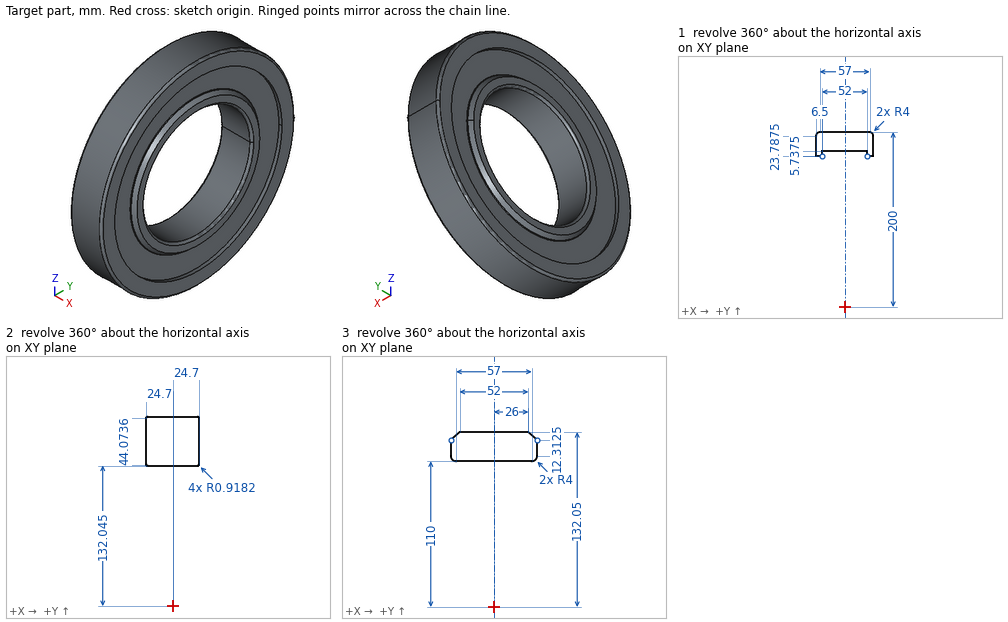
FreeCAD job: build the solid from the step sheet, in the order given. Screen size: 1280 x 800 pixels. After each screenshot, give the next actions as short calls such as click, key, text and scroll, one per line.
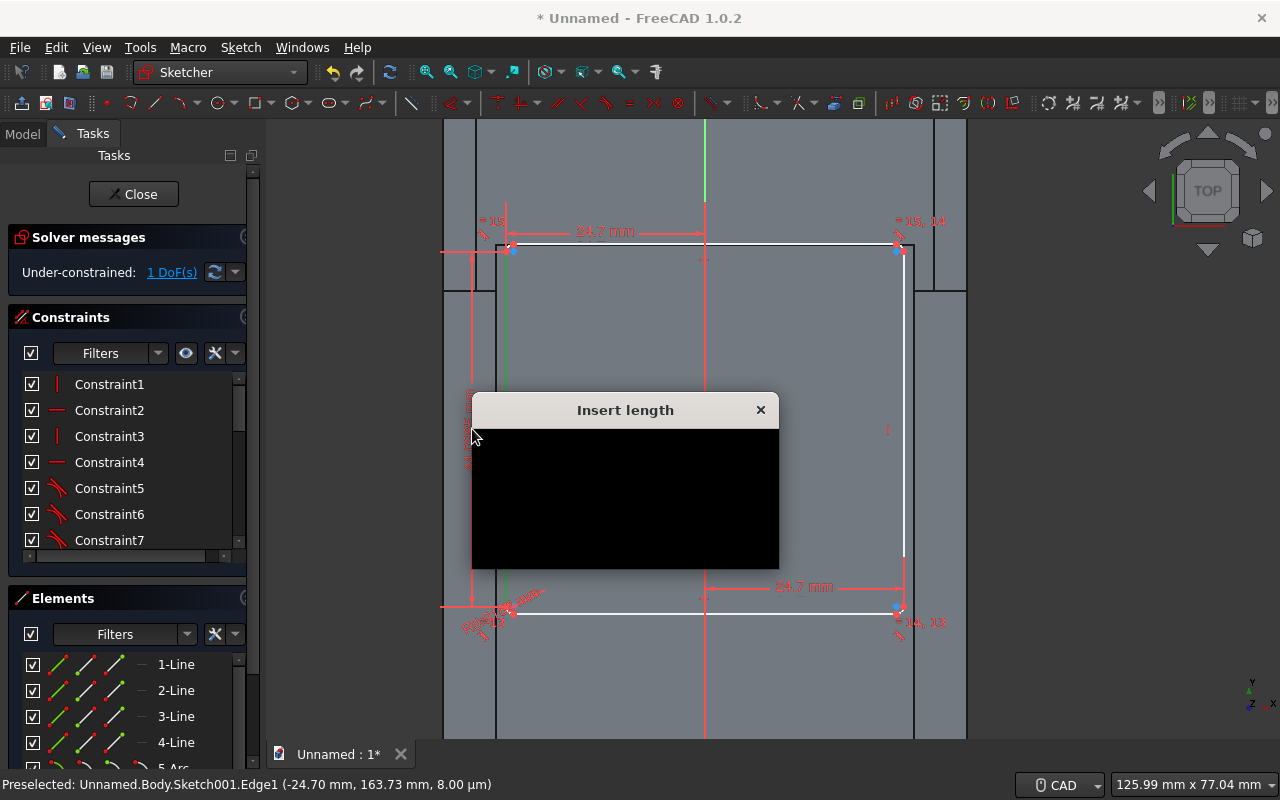
text(44.0736)
key(Return)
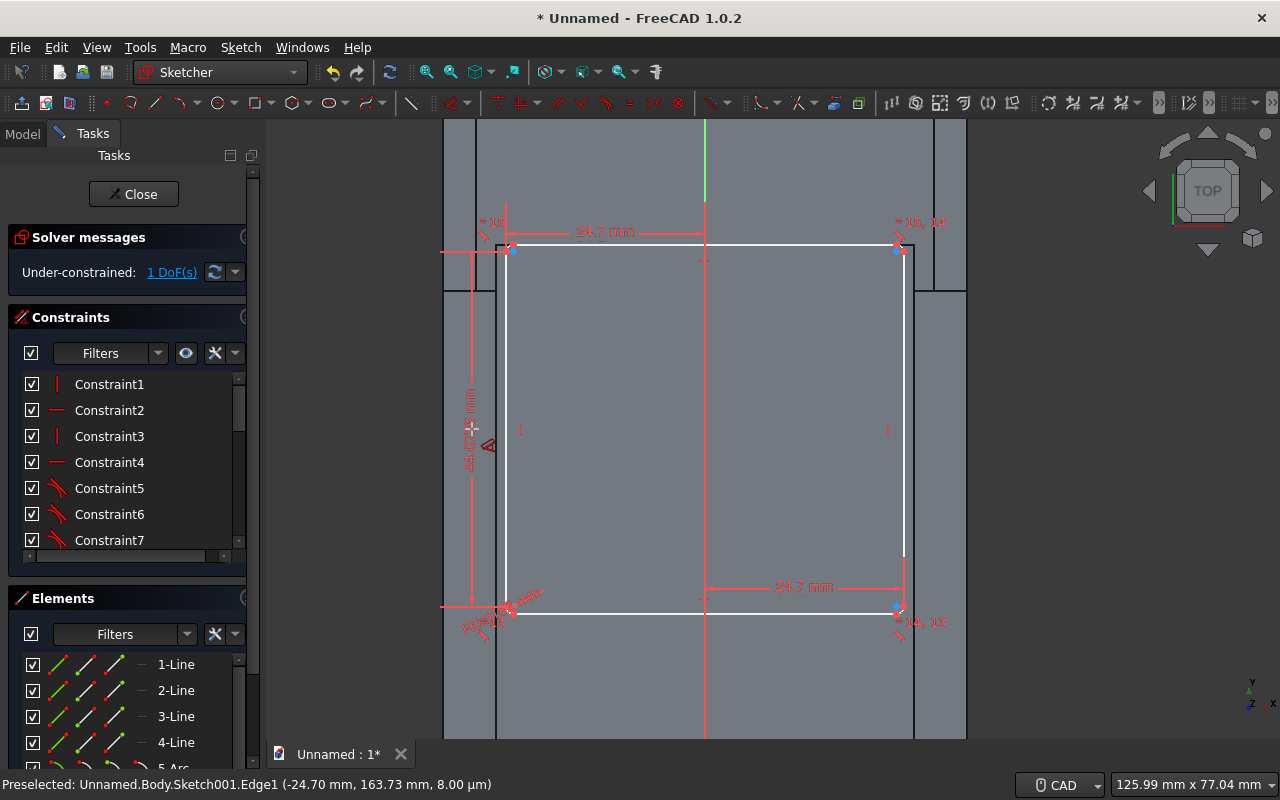
scroll(514, 614, up, 3)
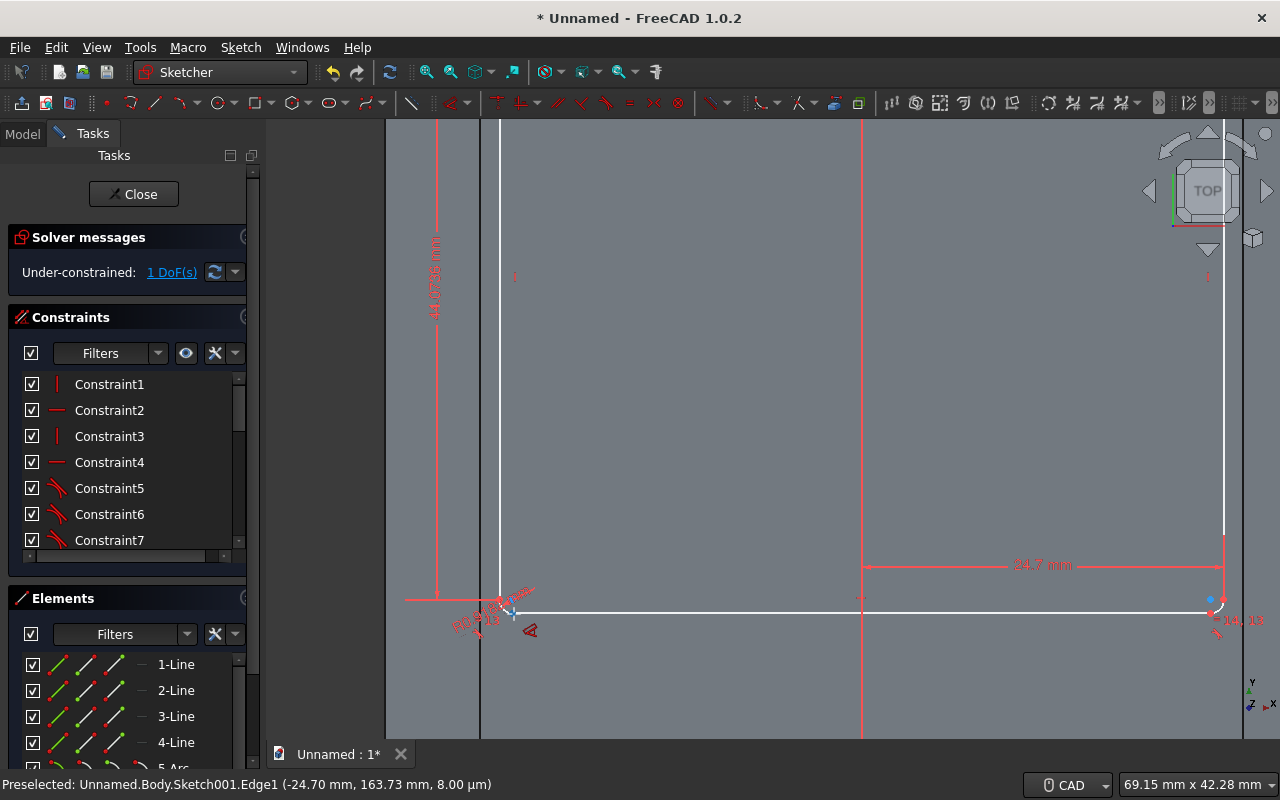
click(513, 613)
click(479, 662)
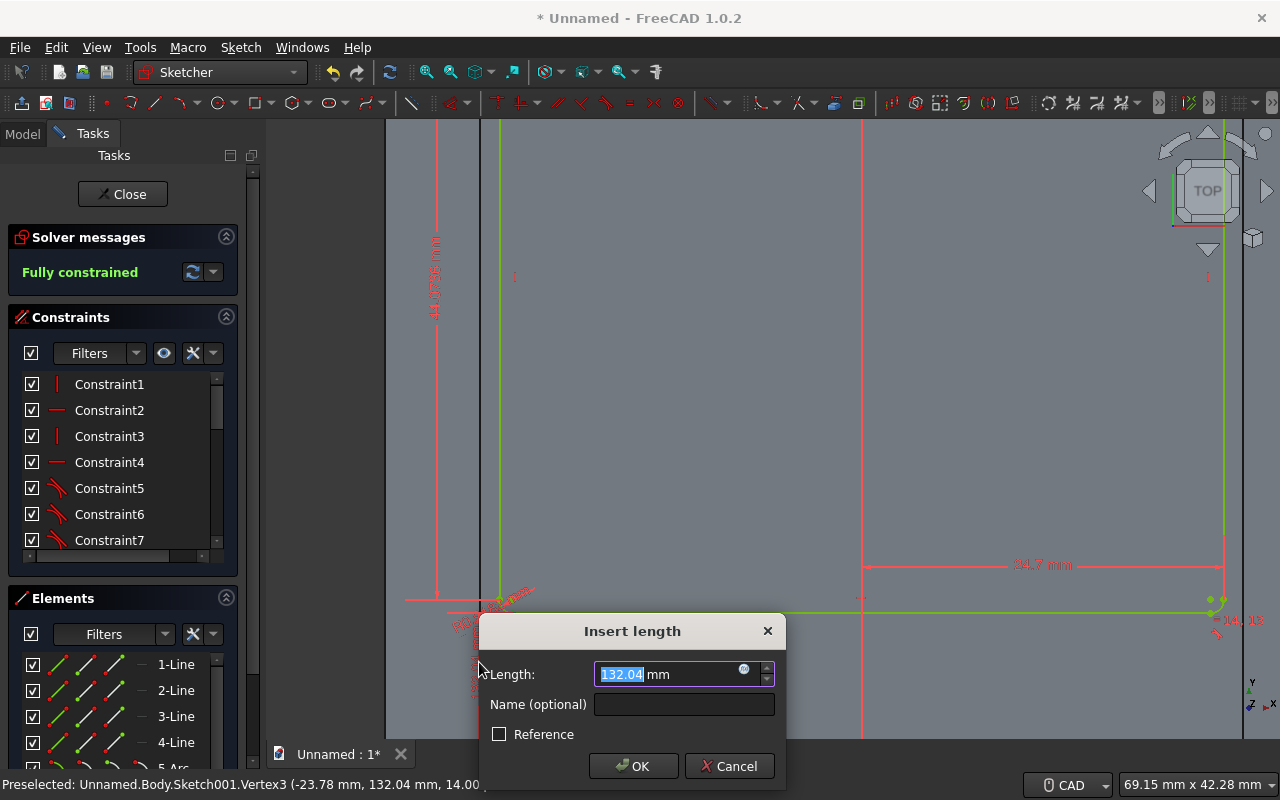
text(132.045)
key(Return)
key(Escape)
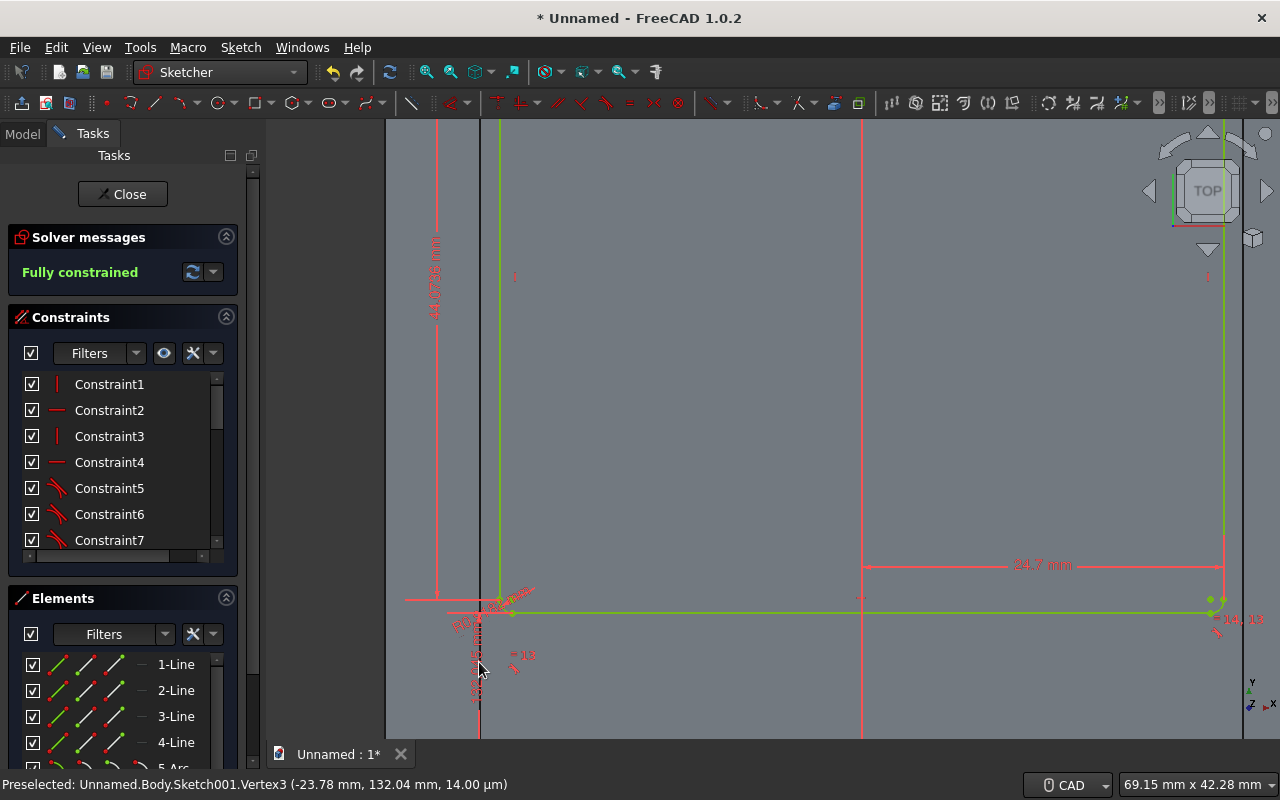
click(123, 194)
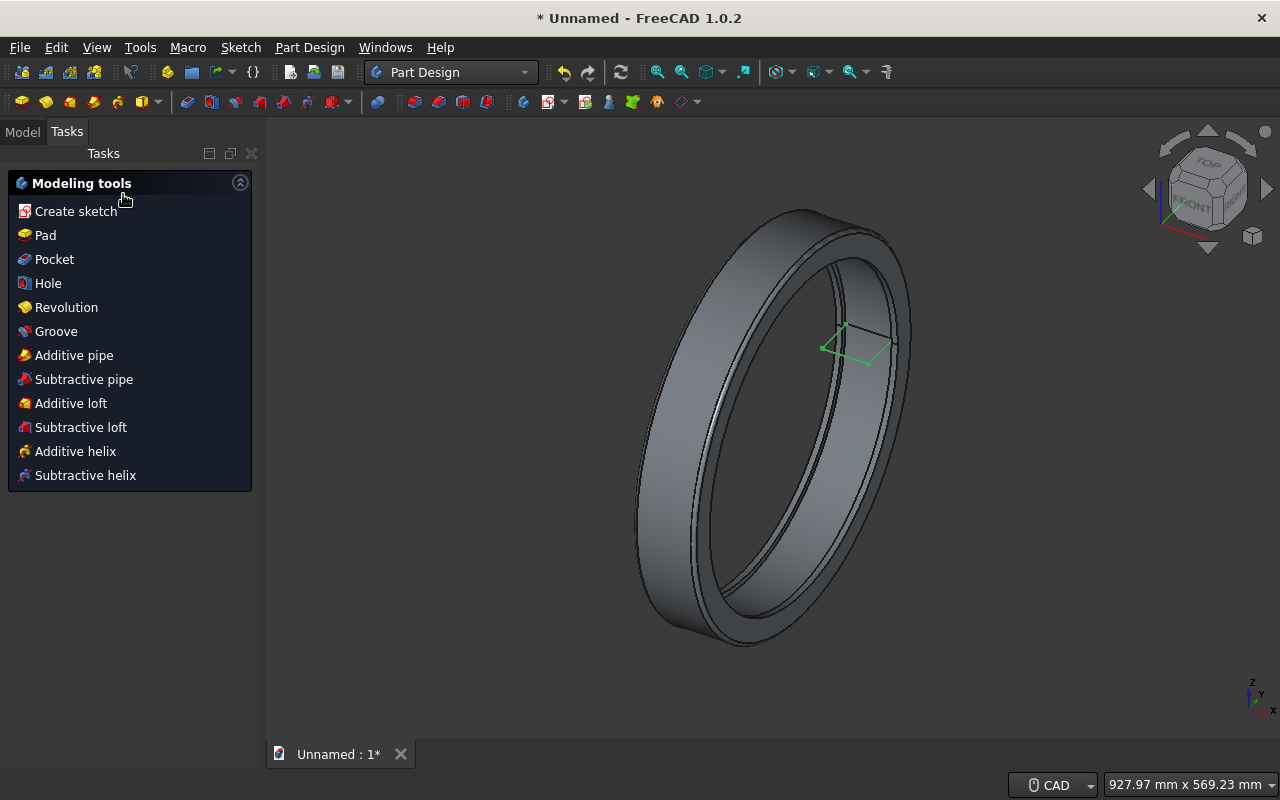
click(46, 102)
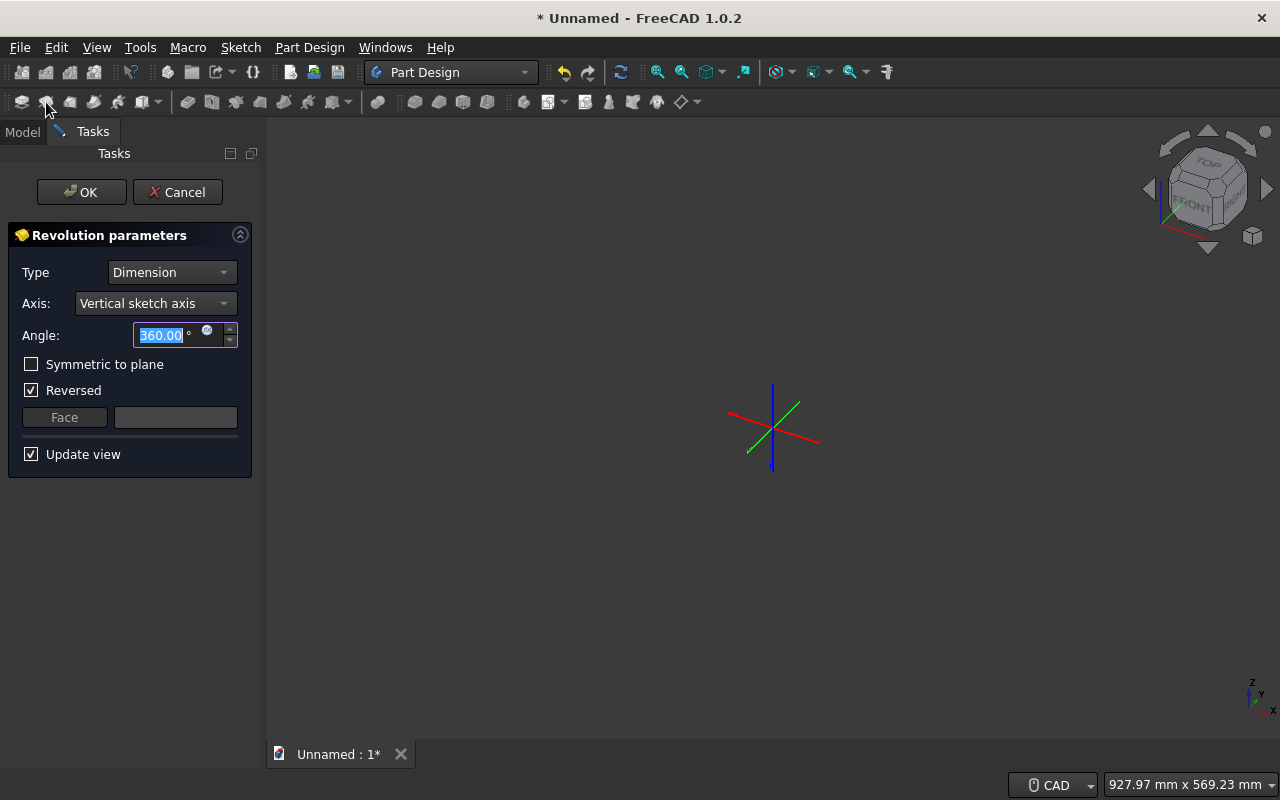
click(156, 304)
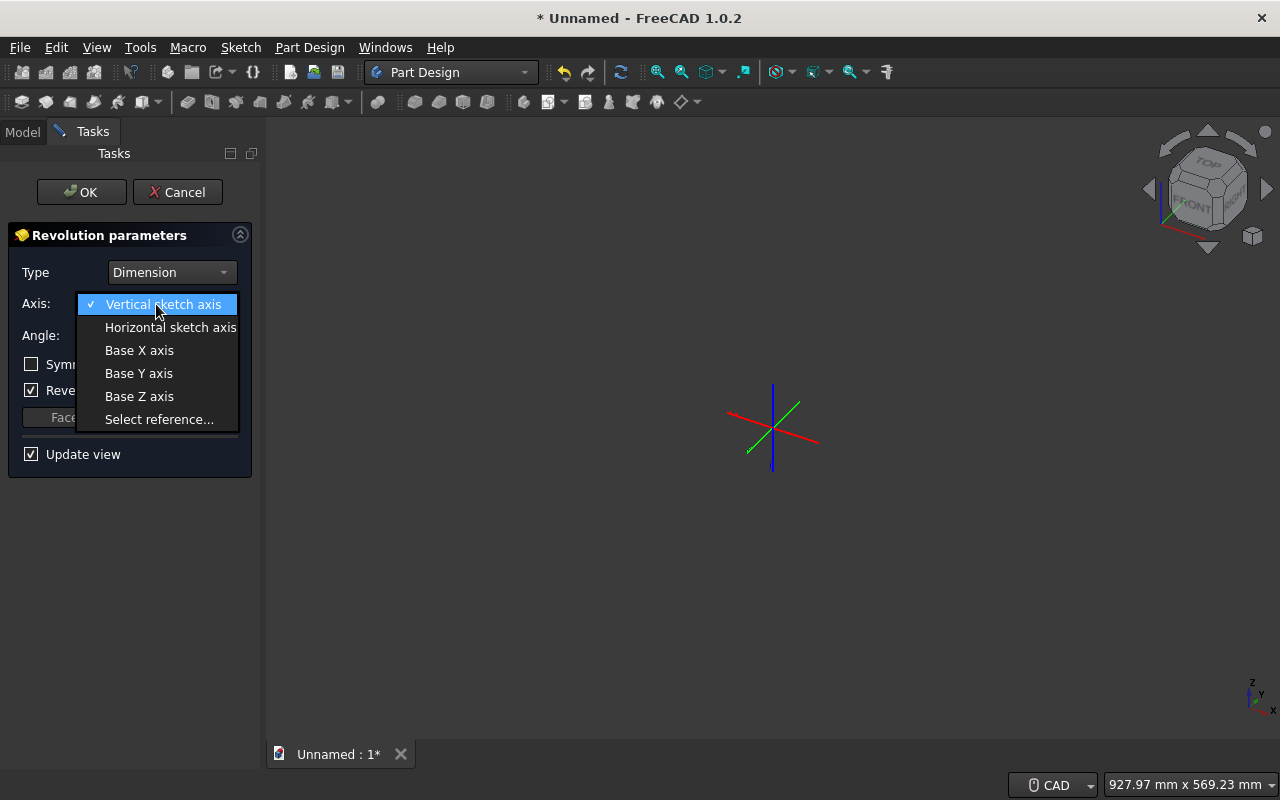
click(156, 328)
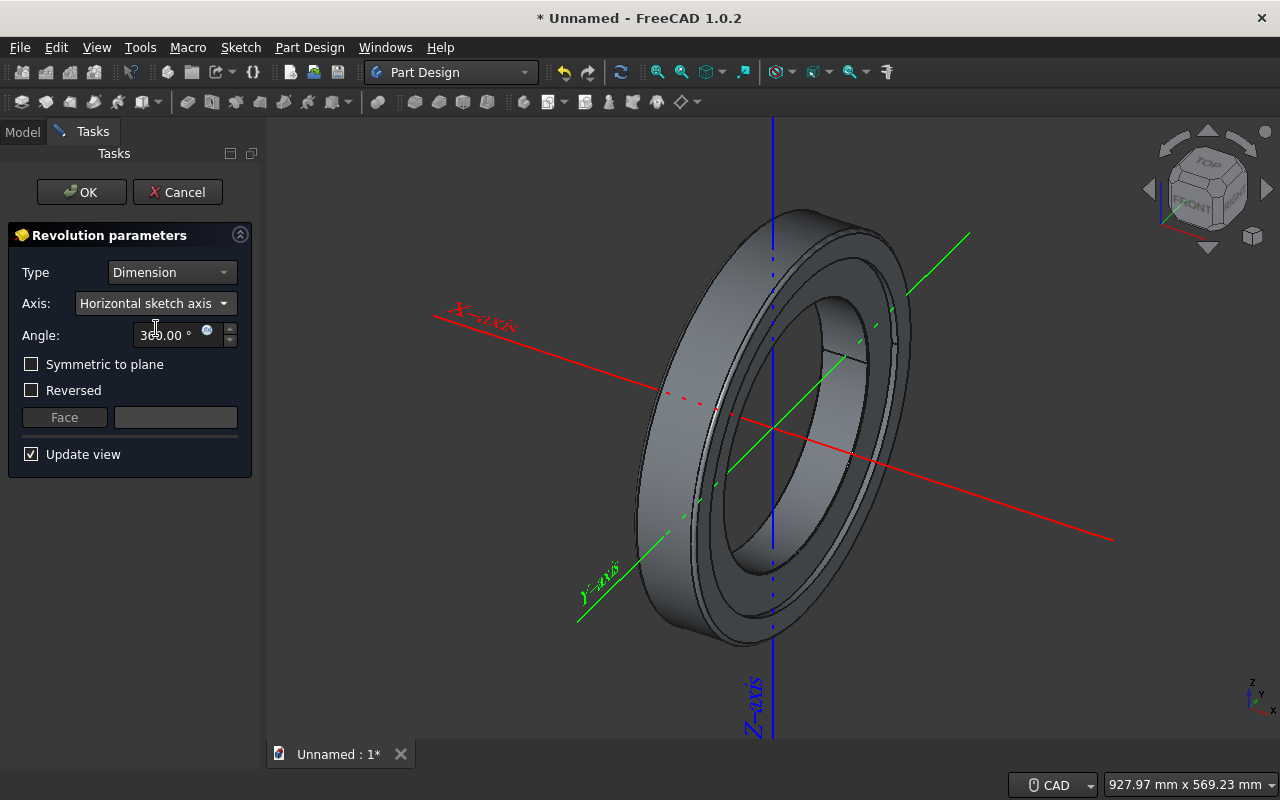
click(82, 192)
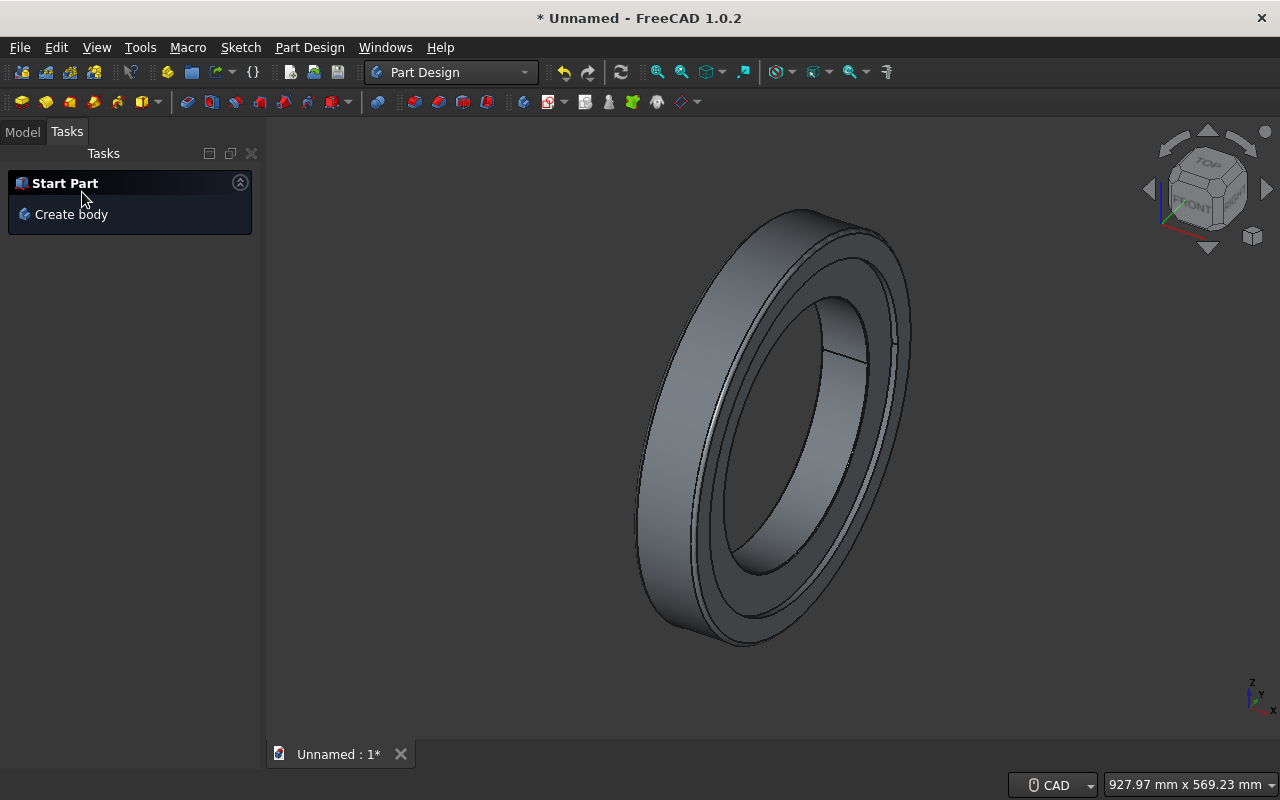
click(548, 102)